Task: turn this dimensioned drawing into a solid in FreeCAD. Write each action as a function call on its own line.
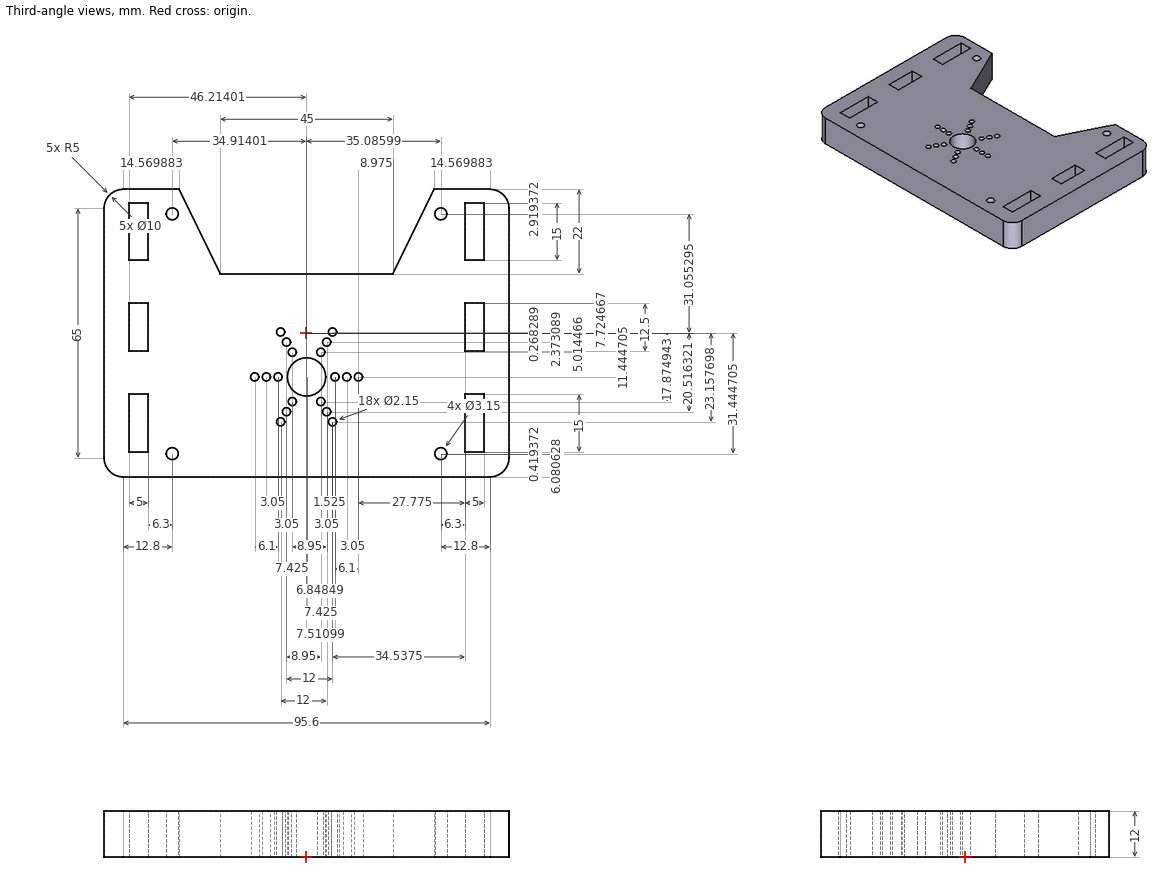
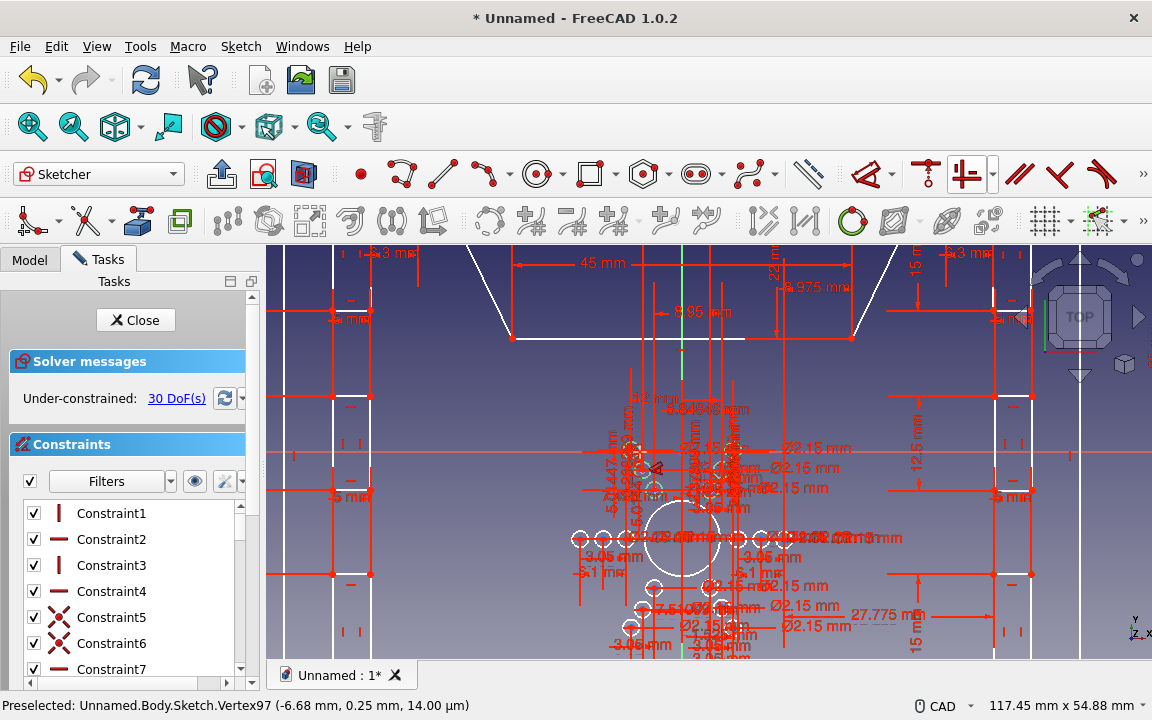
scroll(606, 452, down, 4)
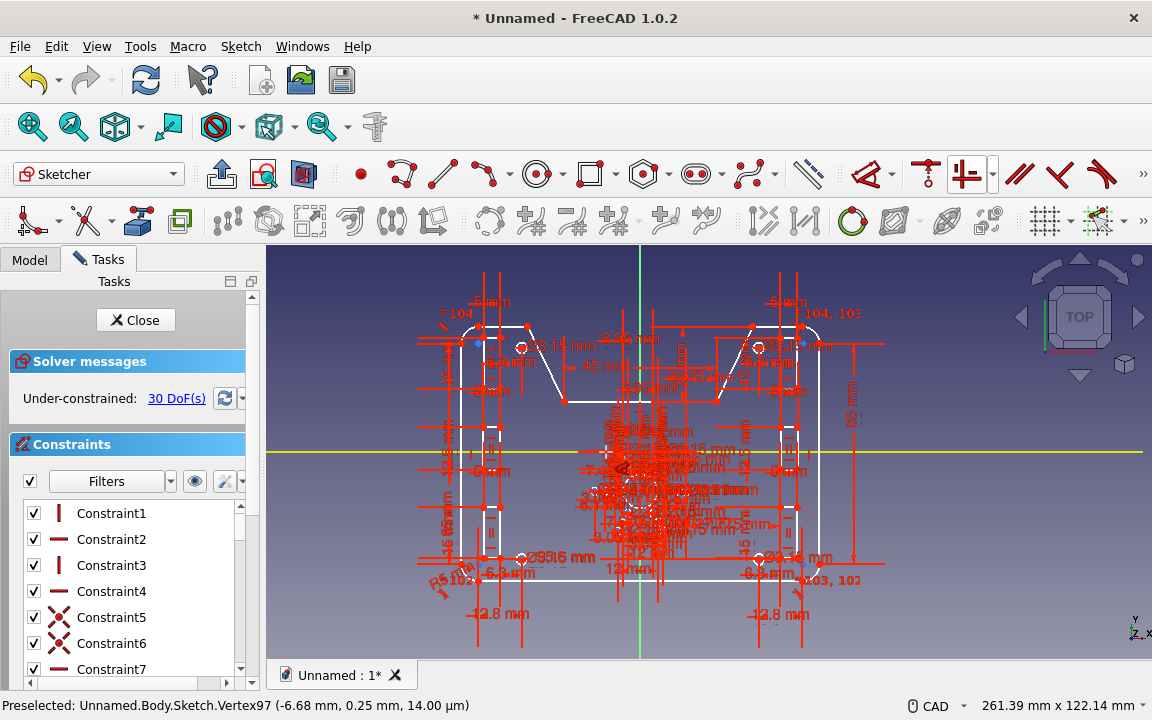
click(759, 348)
click(699, 314)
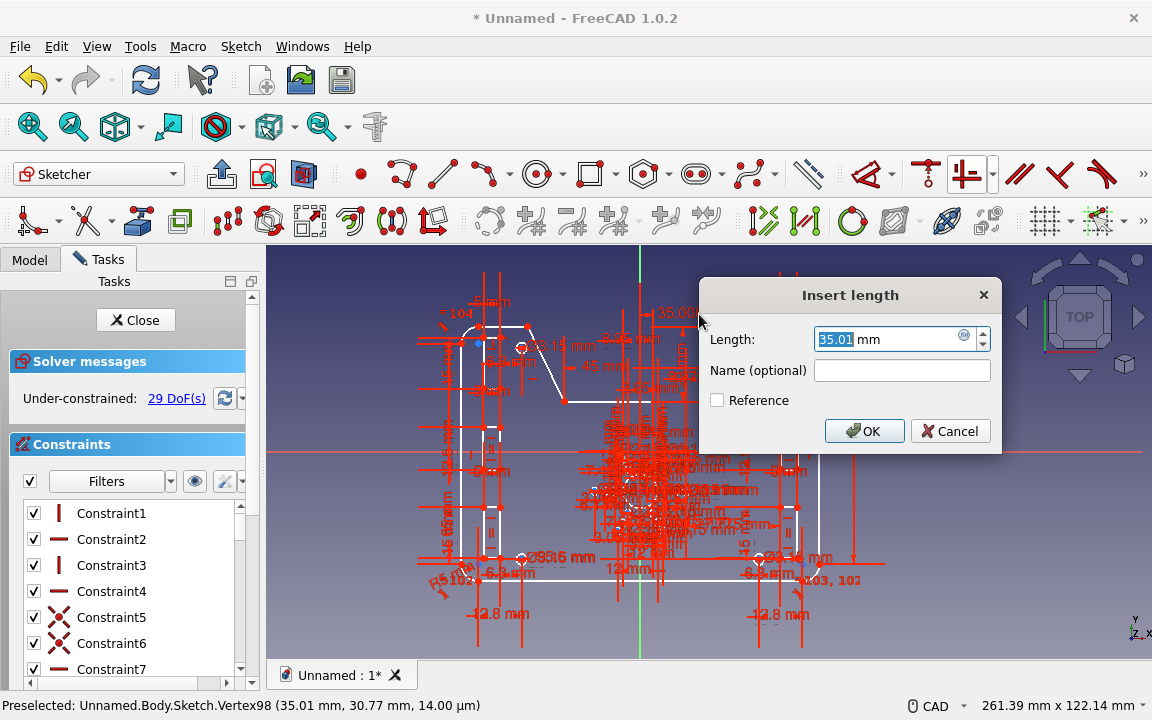
text(35.08599)
key(Return)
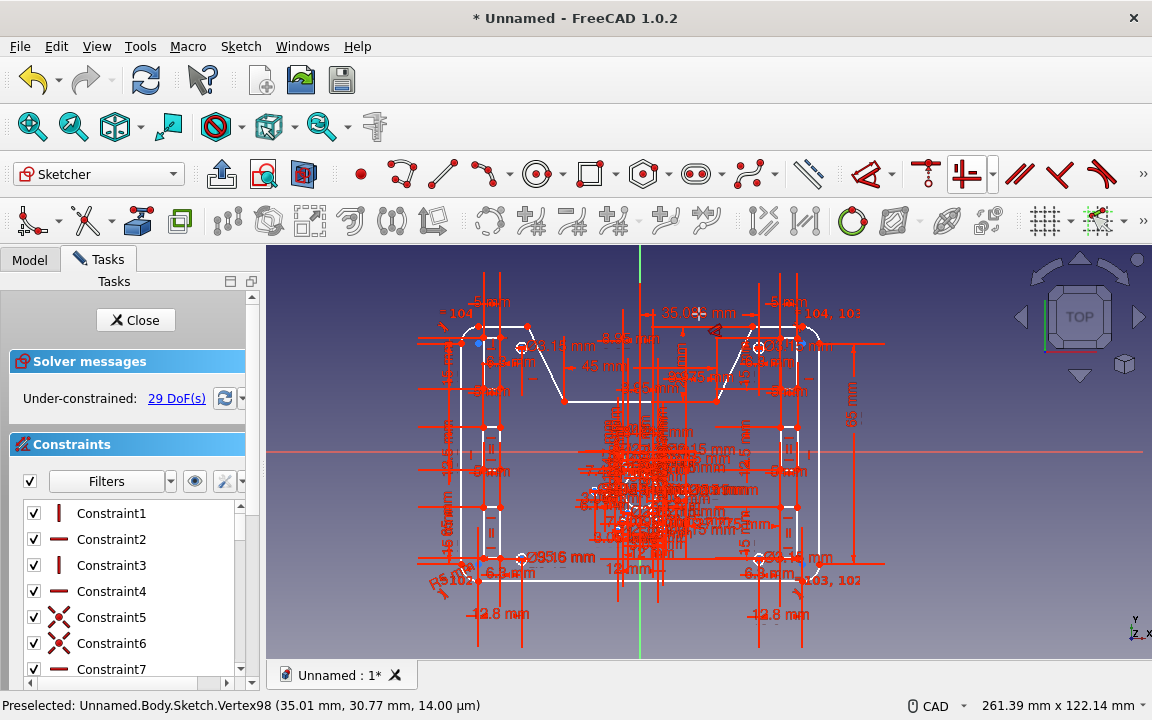
click(522, 348)
click(581, 314)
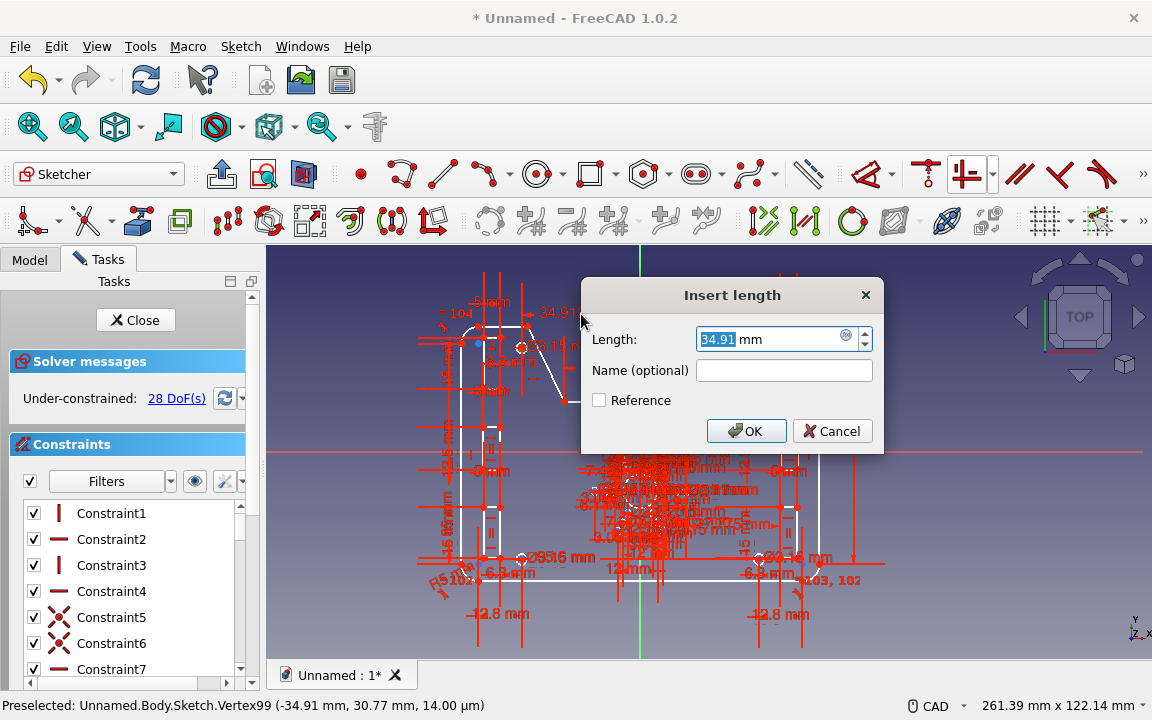
text(34.91401)
key(Return)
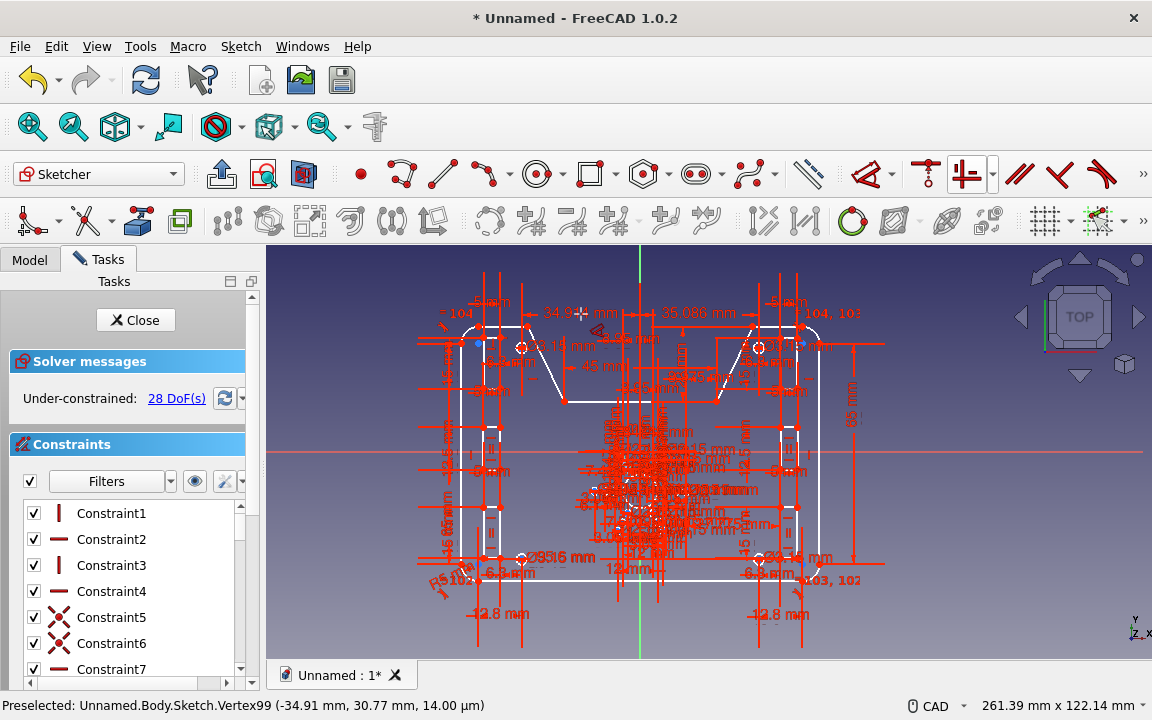
click(781, 470)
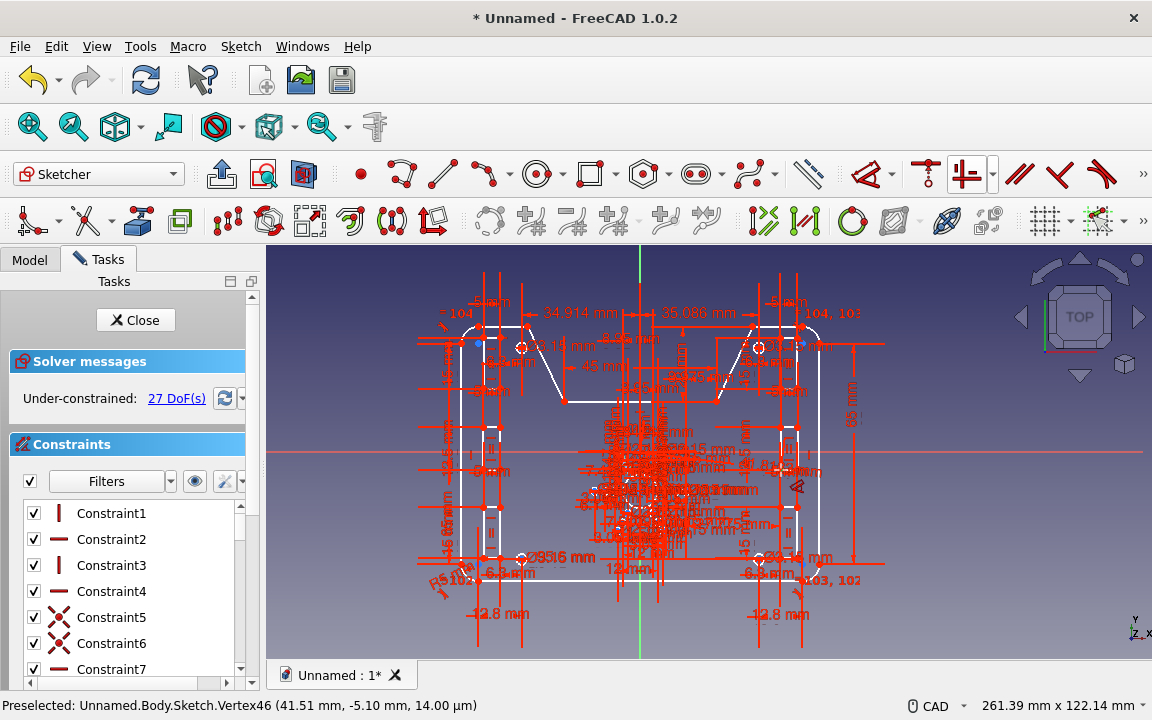
click(663, 531)
click(749, 436)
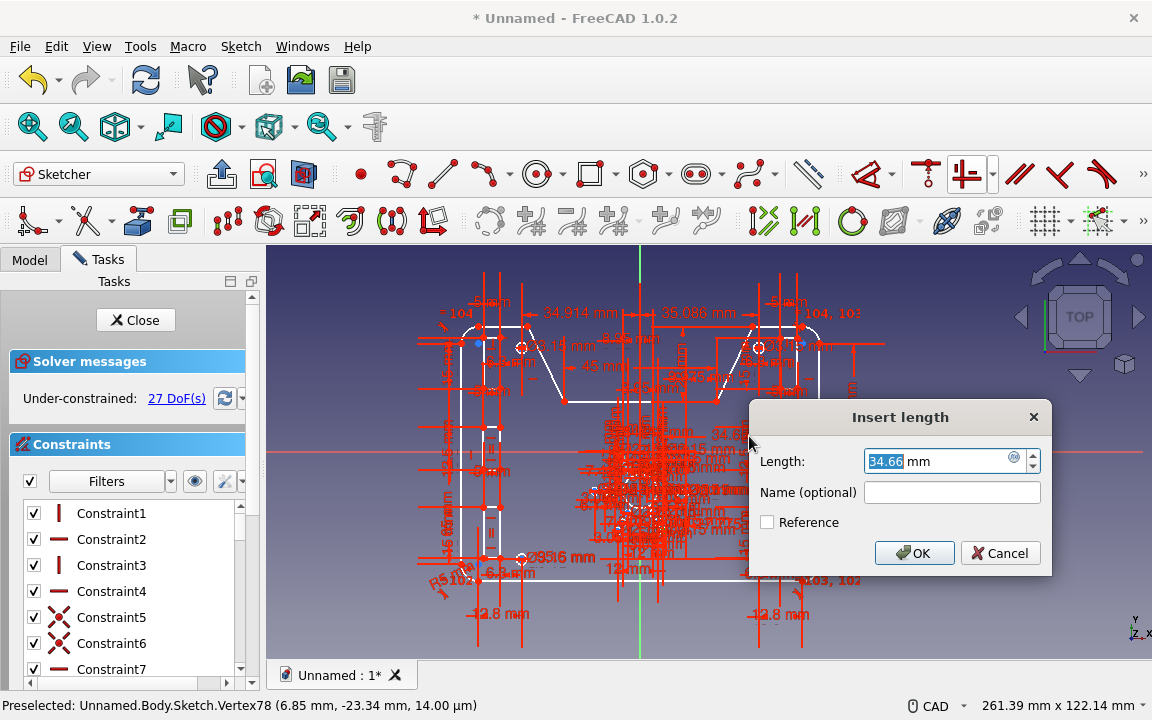
text(34.5375)
key(Return)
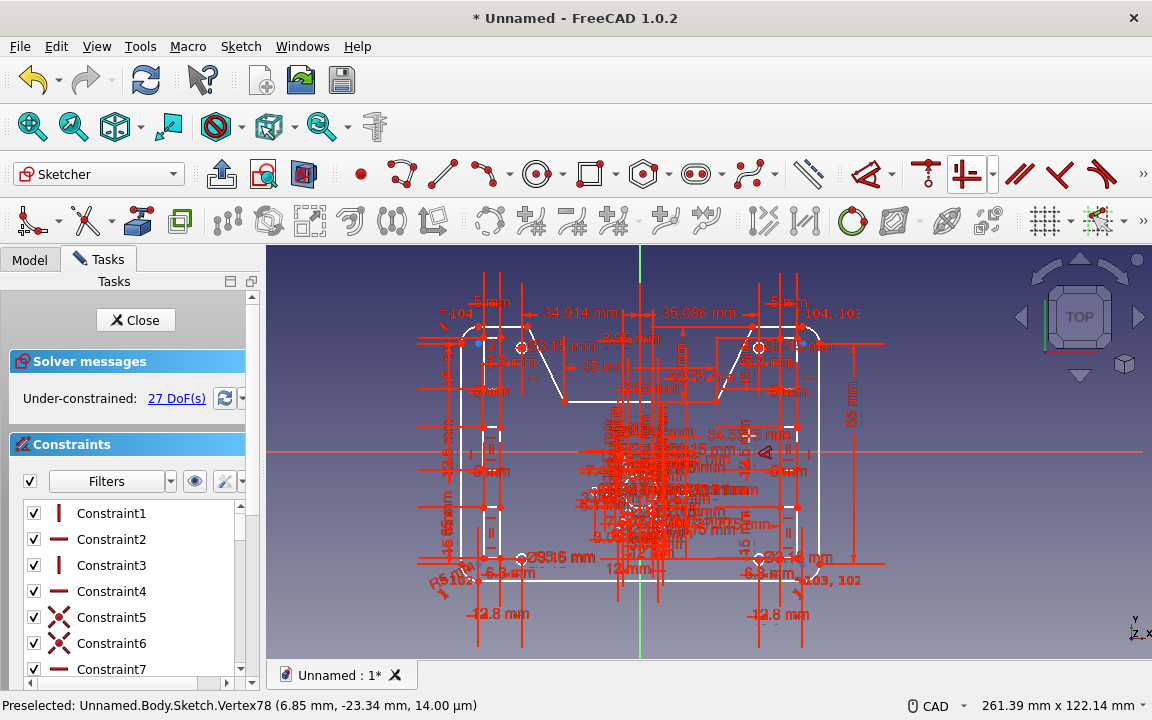
scroll(788, 327, up, 2)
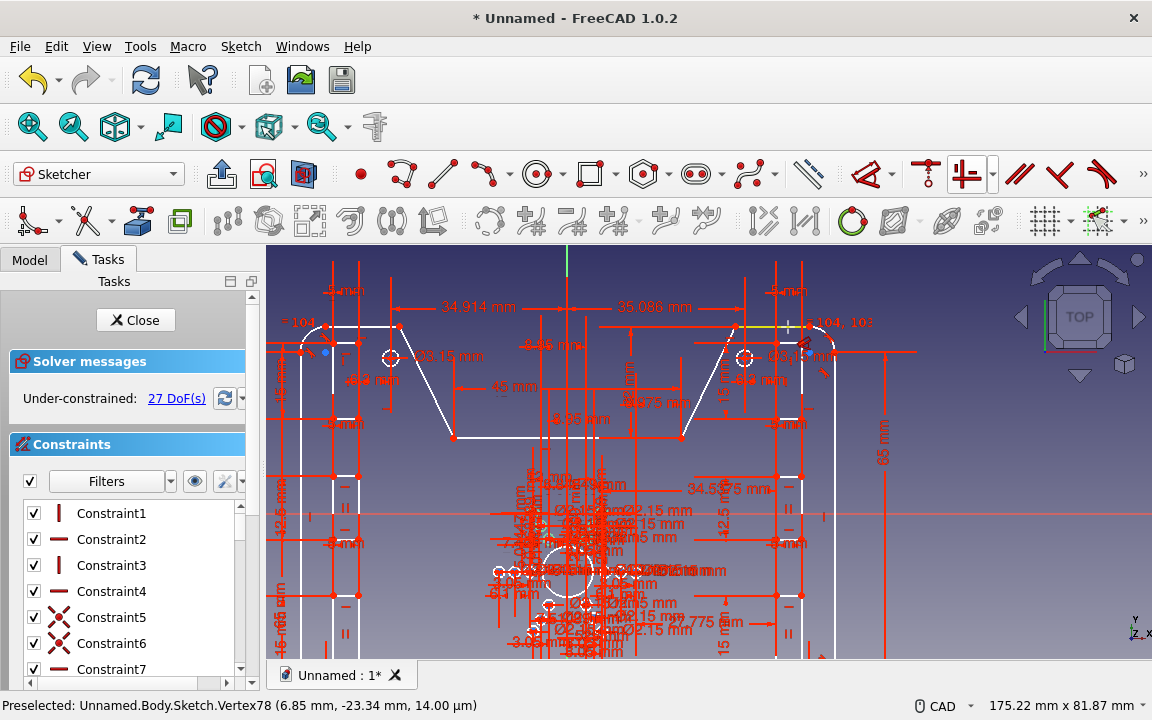
click(787, 327)
click(772, 293)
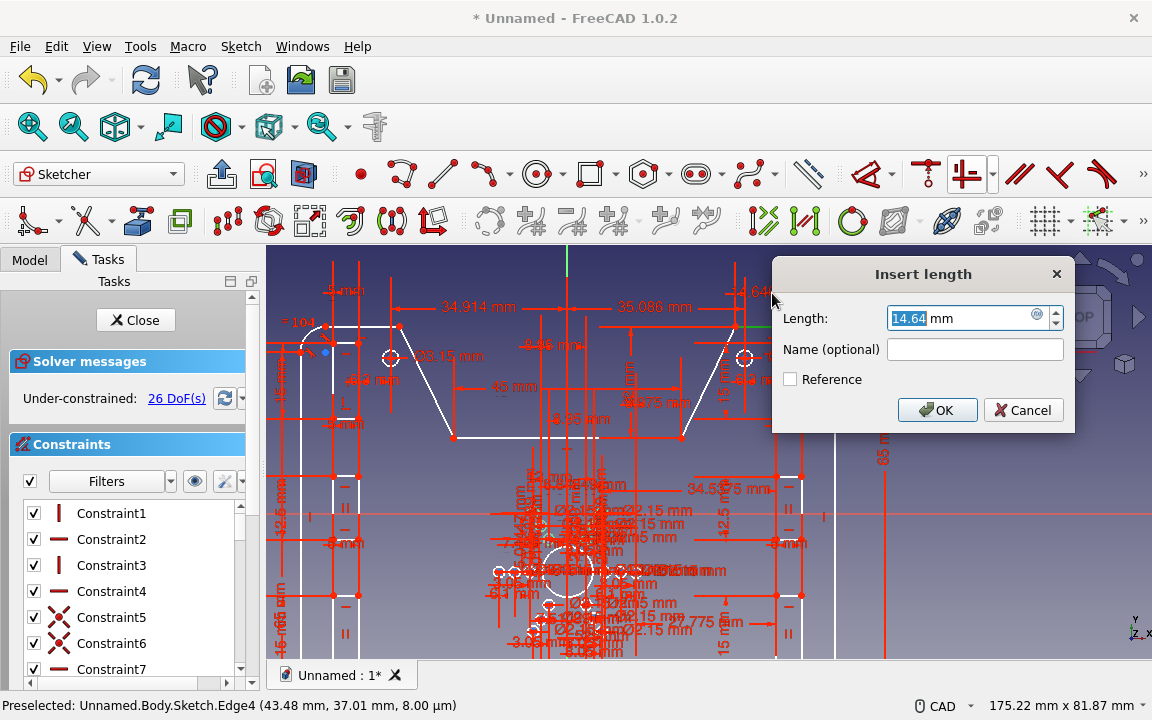
text(14.569883)
key(Return)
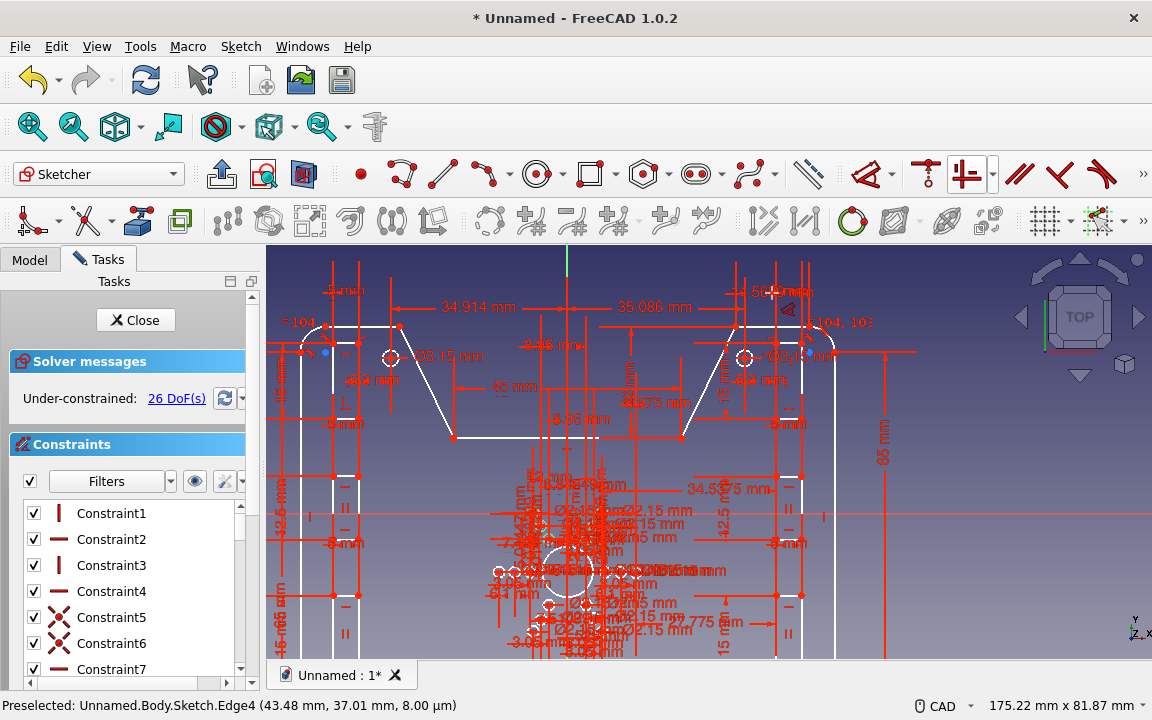
click(377, 327)
click(363, 293)